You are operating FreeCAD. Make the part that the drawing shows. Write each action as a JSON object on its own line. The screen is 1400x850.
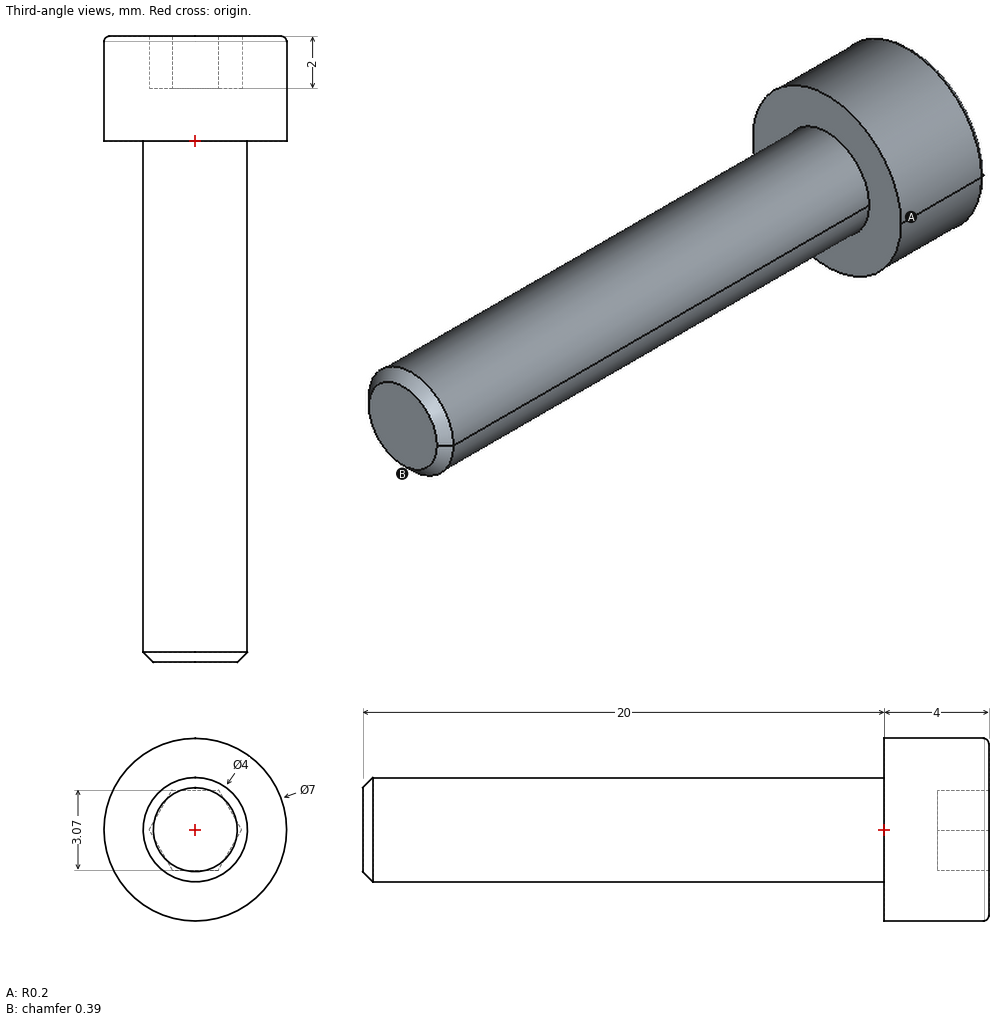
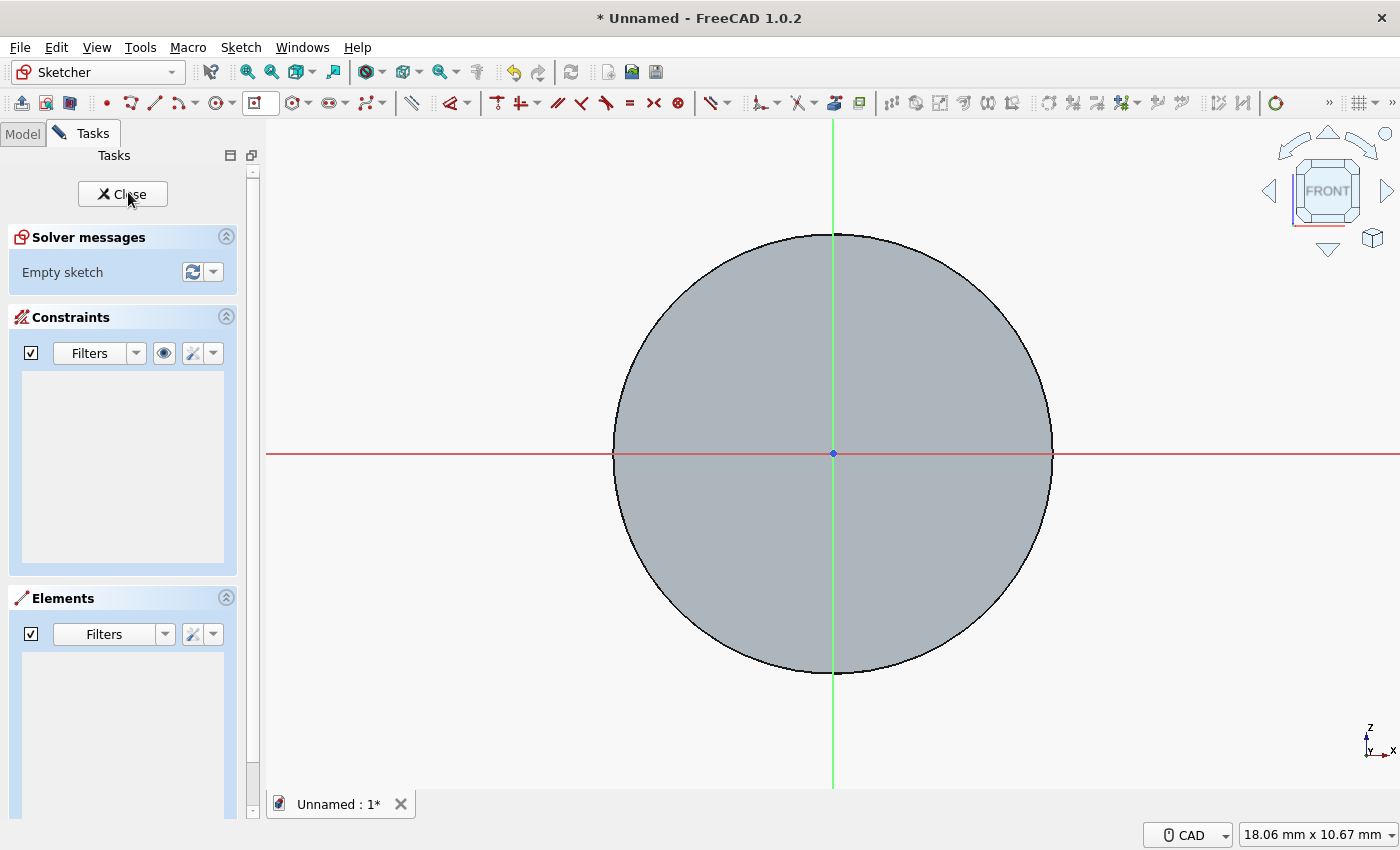
{"action": "scroll", "coordinate": [916, 454], "scroll_direction": "up", "scroll_amount": 3}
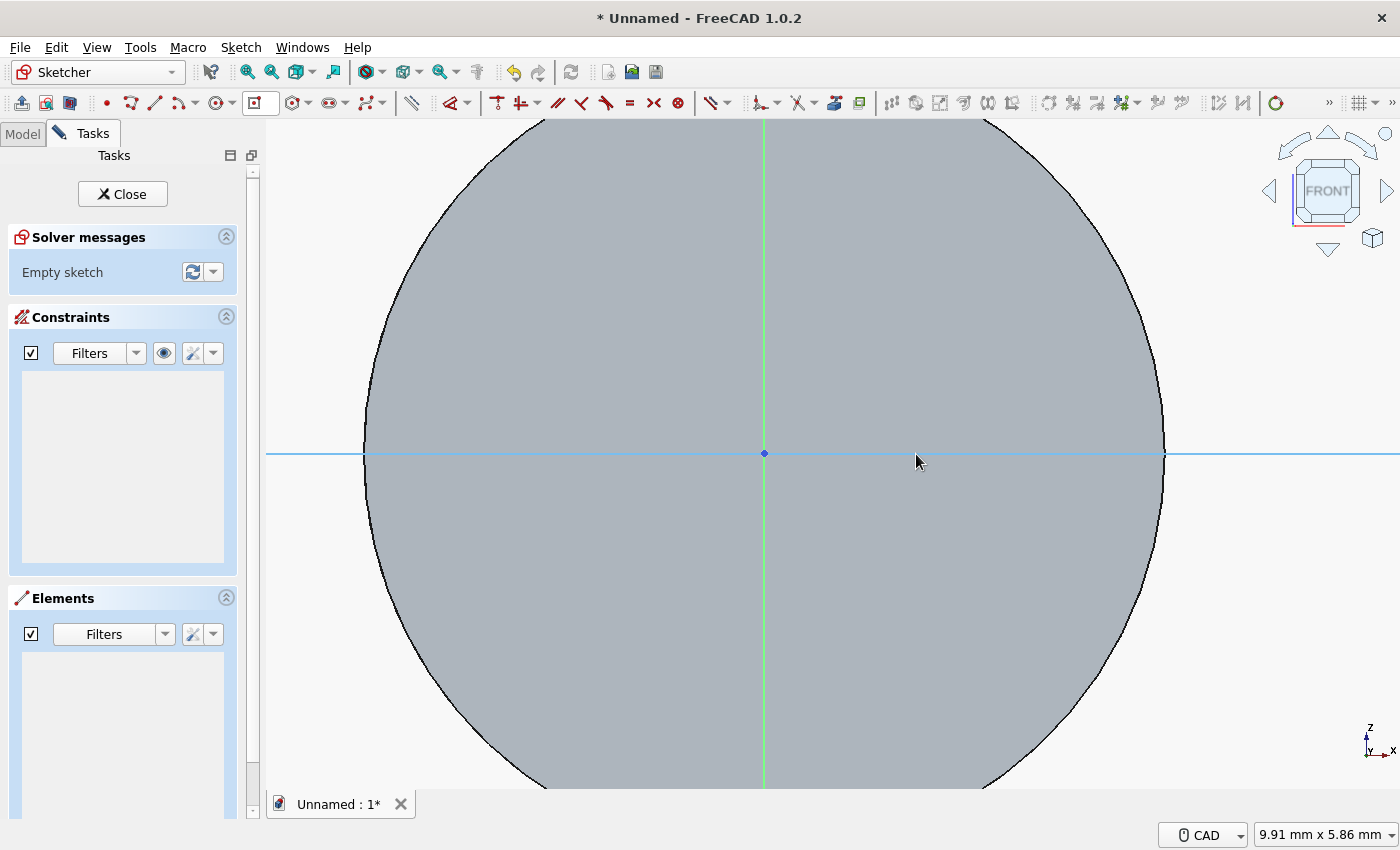
{"action": "key", "text": "g c"}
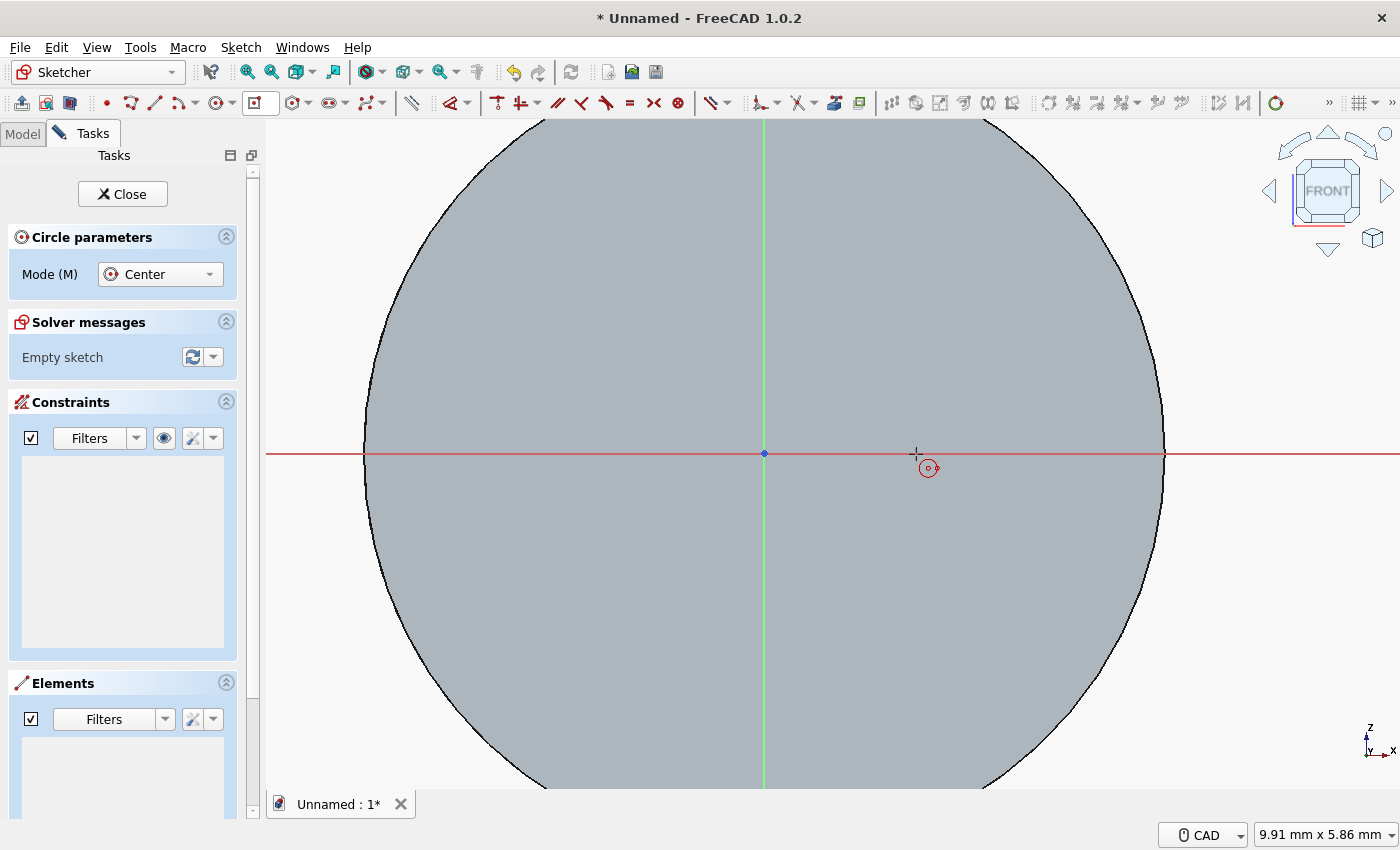
{"action": "left_click", "coordinate": [764, 454]}
{"action": "left_click", "coordinate": [926, 292]}
{"action": "key", "text": "Escape"}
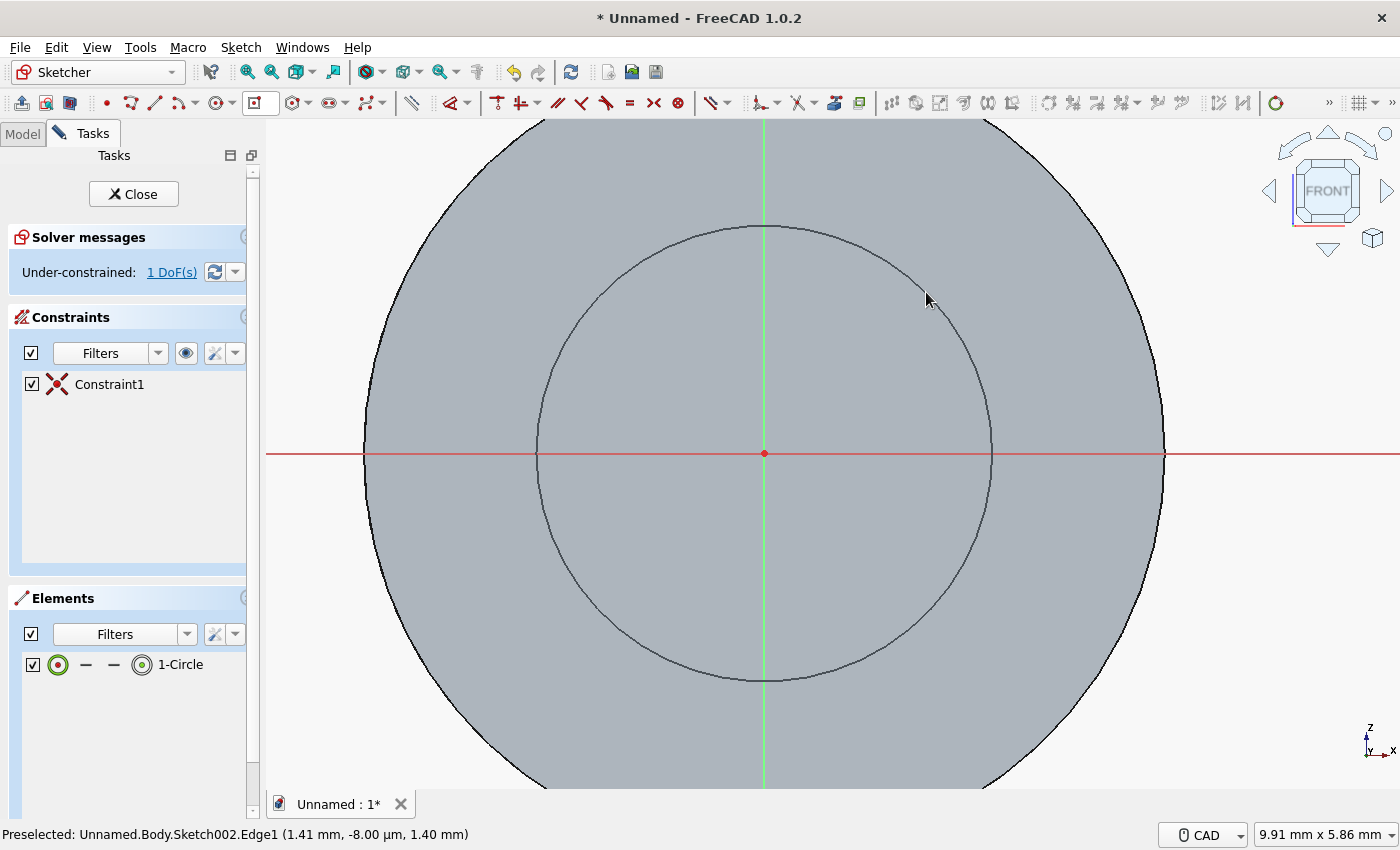
{"action": "key", "text": "d"}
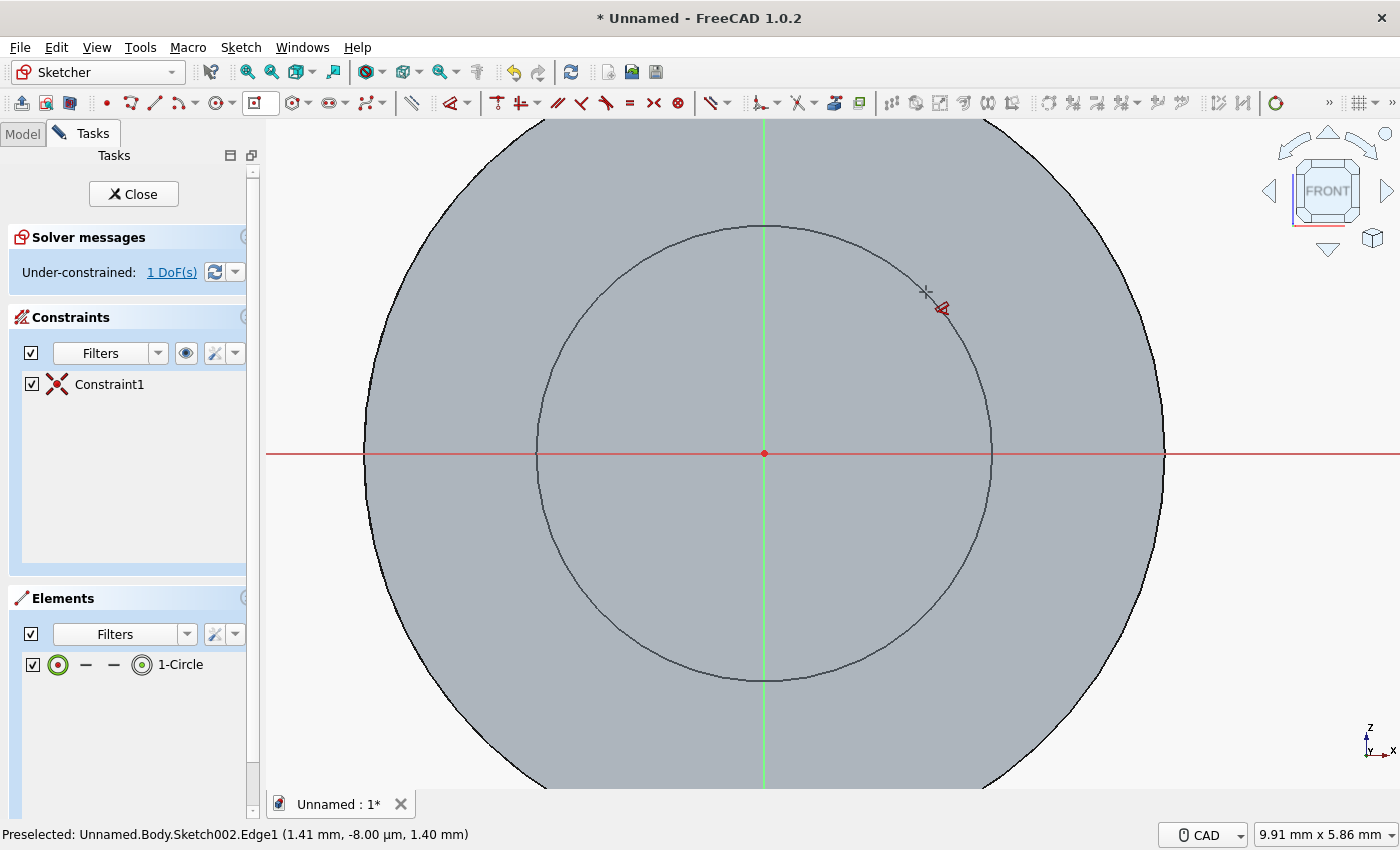
{"action": "left_click", "coordinate": [925, 292]}
{"action": "left_click", "coordinate": [948, 269]}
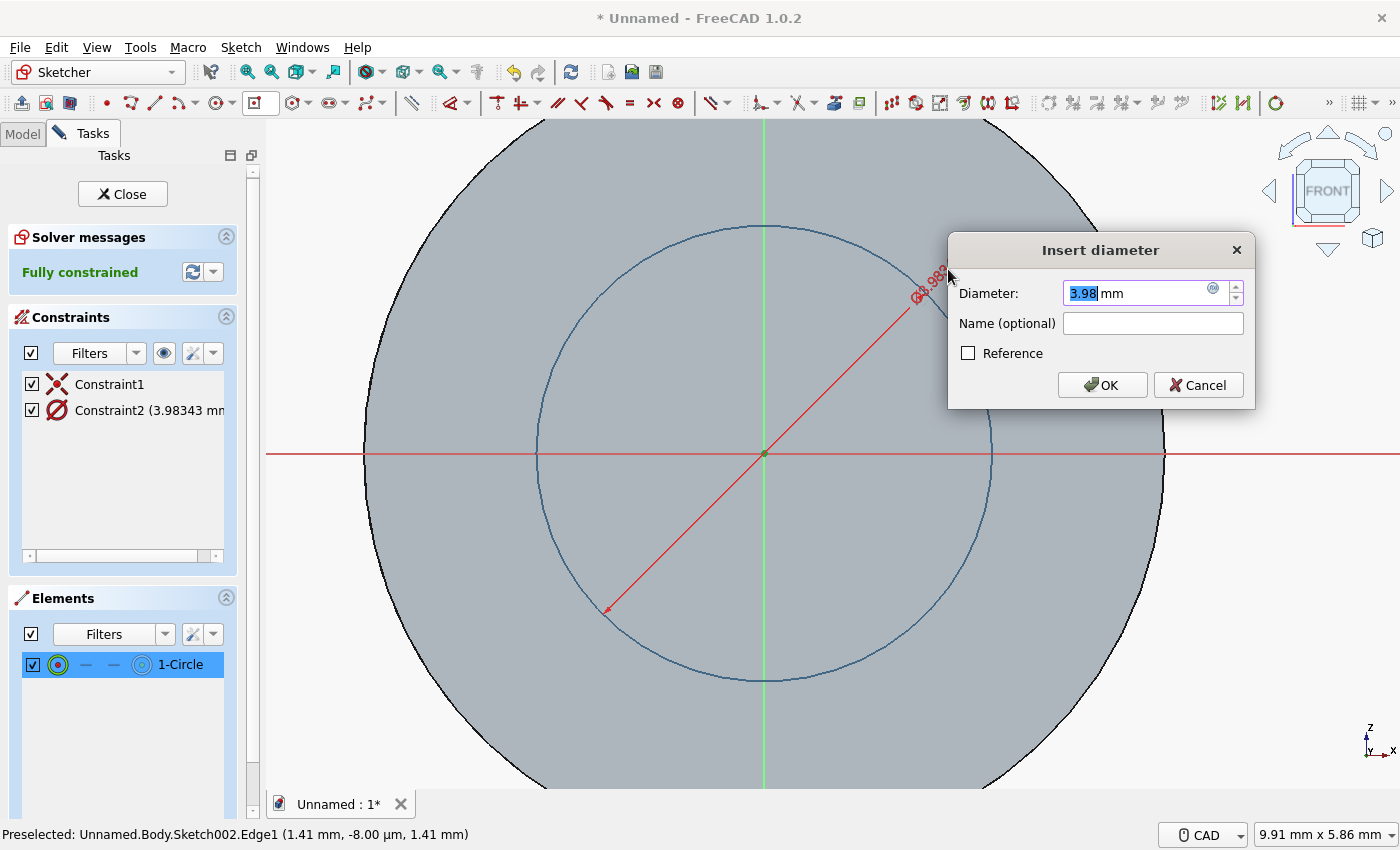
{"action": "type", "text": "4"}
{"action": "key", "text": "Return"}
{"action": "key", "text": "Escape"}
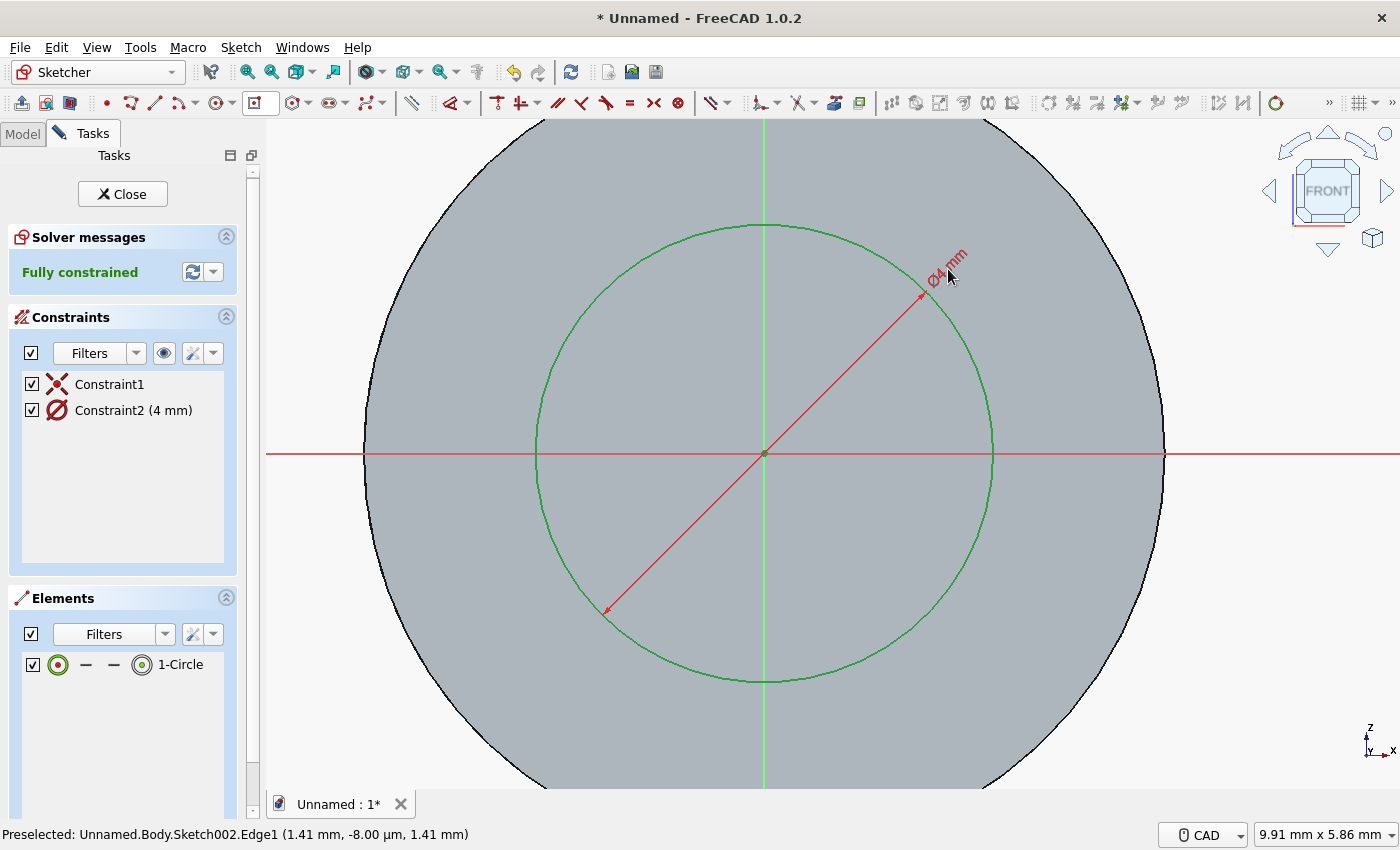
{"action": "left_click", "coordinate": [123, 194]}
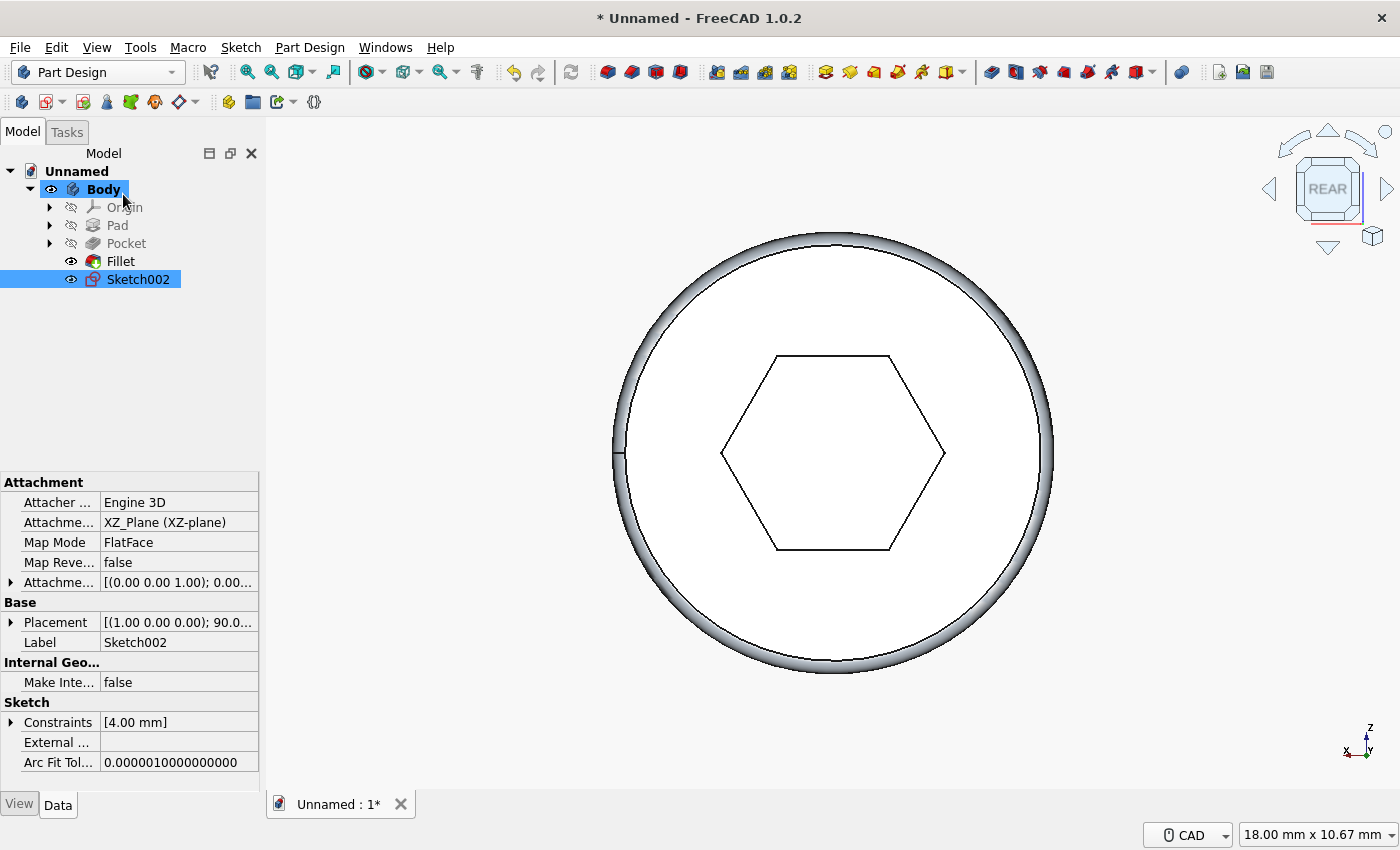
{"action": "left_click", "coordinate": [826, 72]}